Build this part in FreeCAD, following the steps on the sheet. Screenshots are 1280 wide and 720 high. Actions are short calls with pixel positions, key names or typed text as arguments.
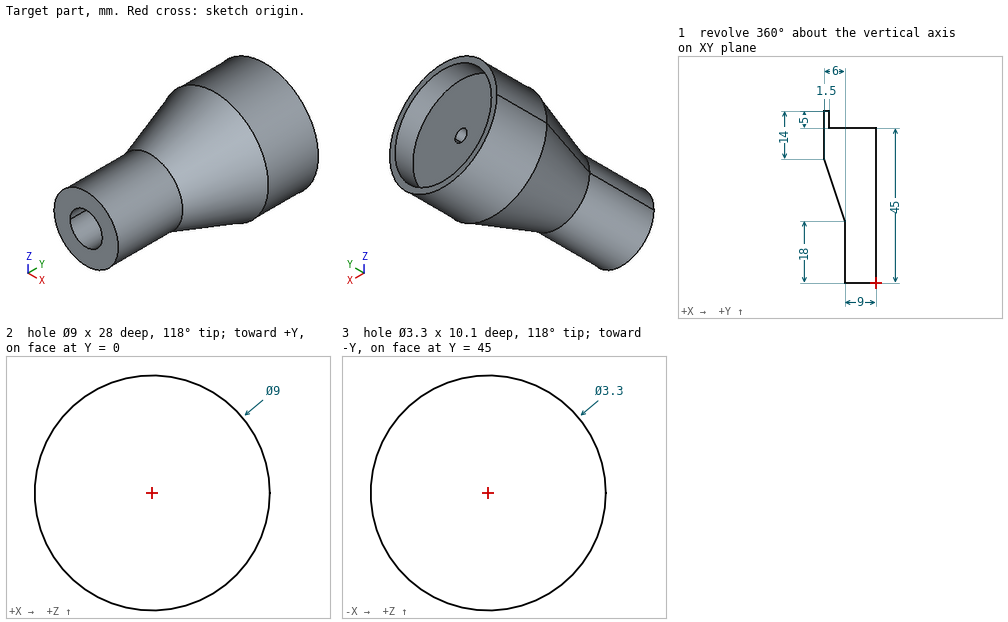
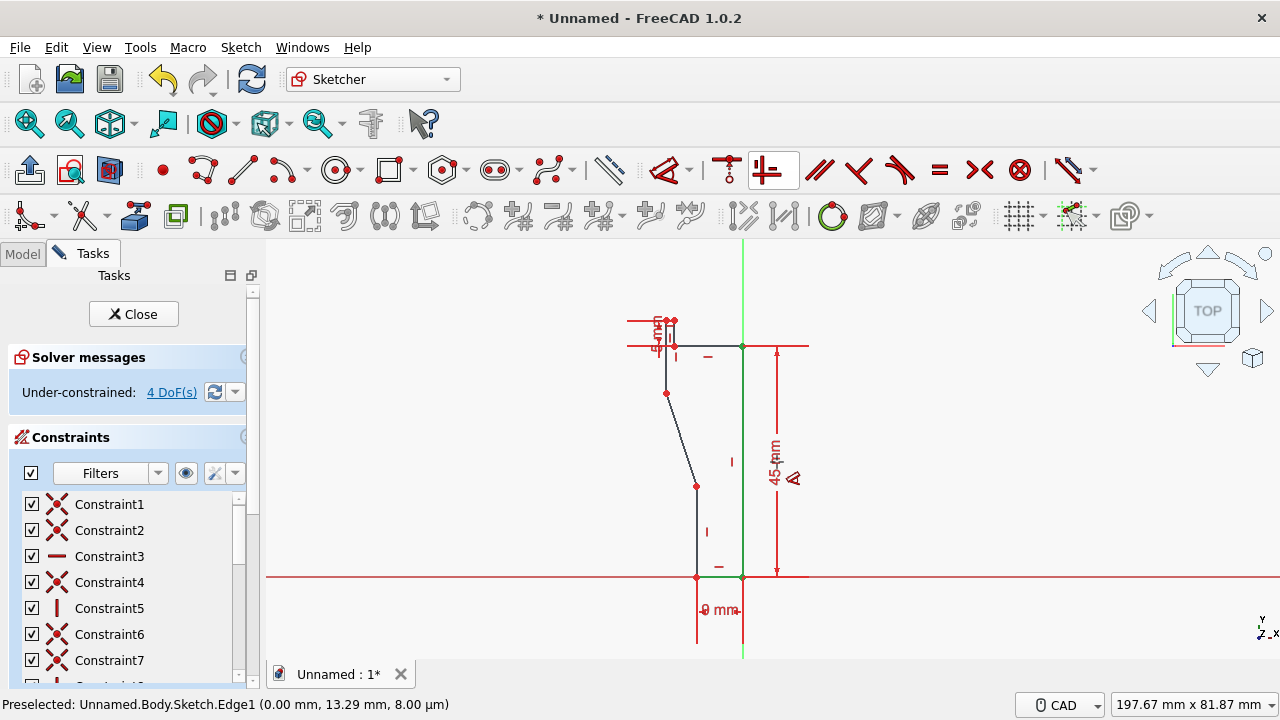
click(666, 371)
click(632, 357)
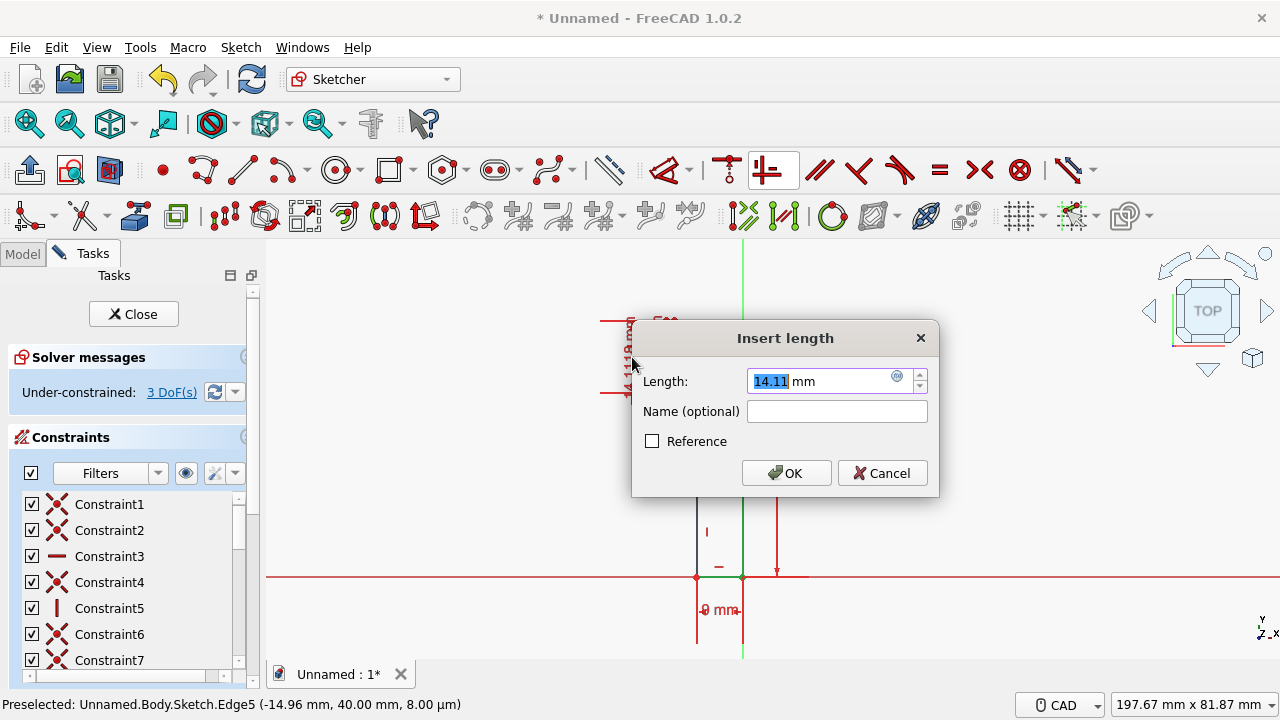
text(14)
key(Return)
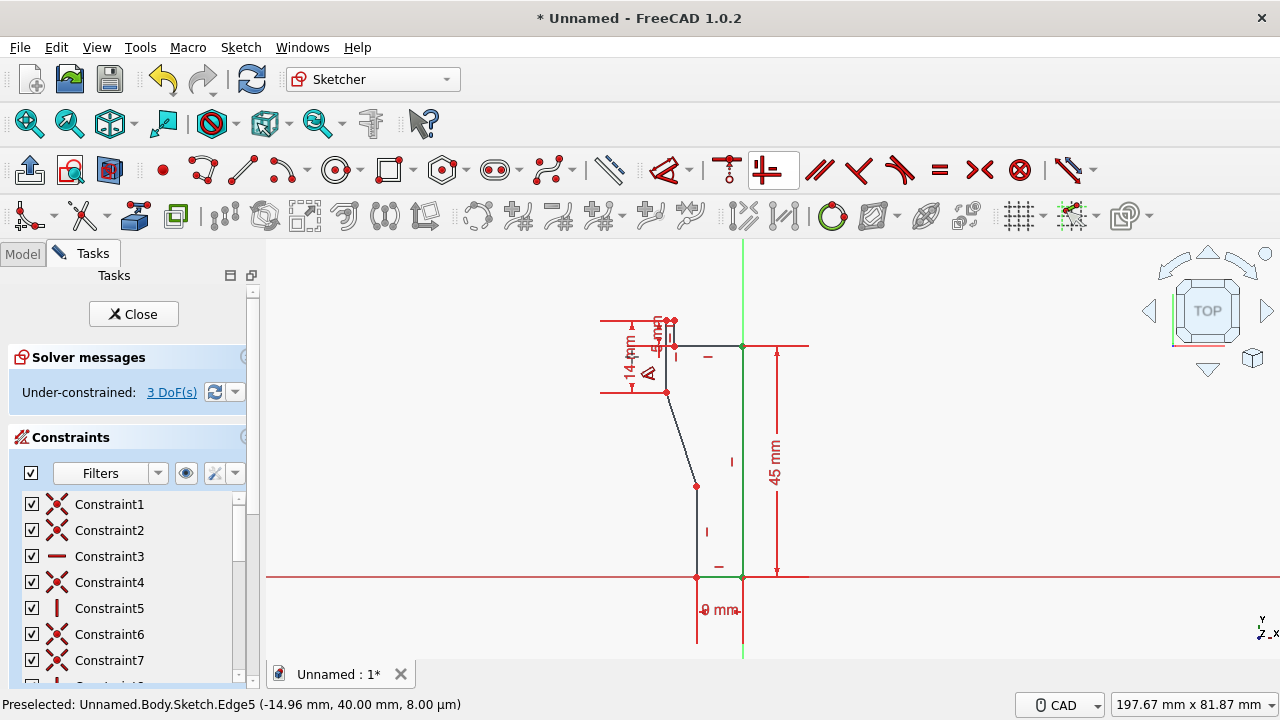
click(697, 513)
click(663, 532)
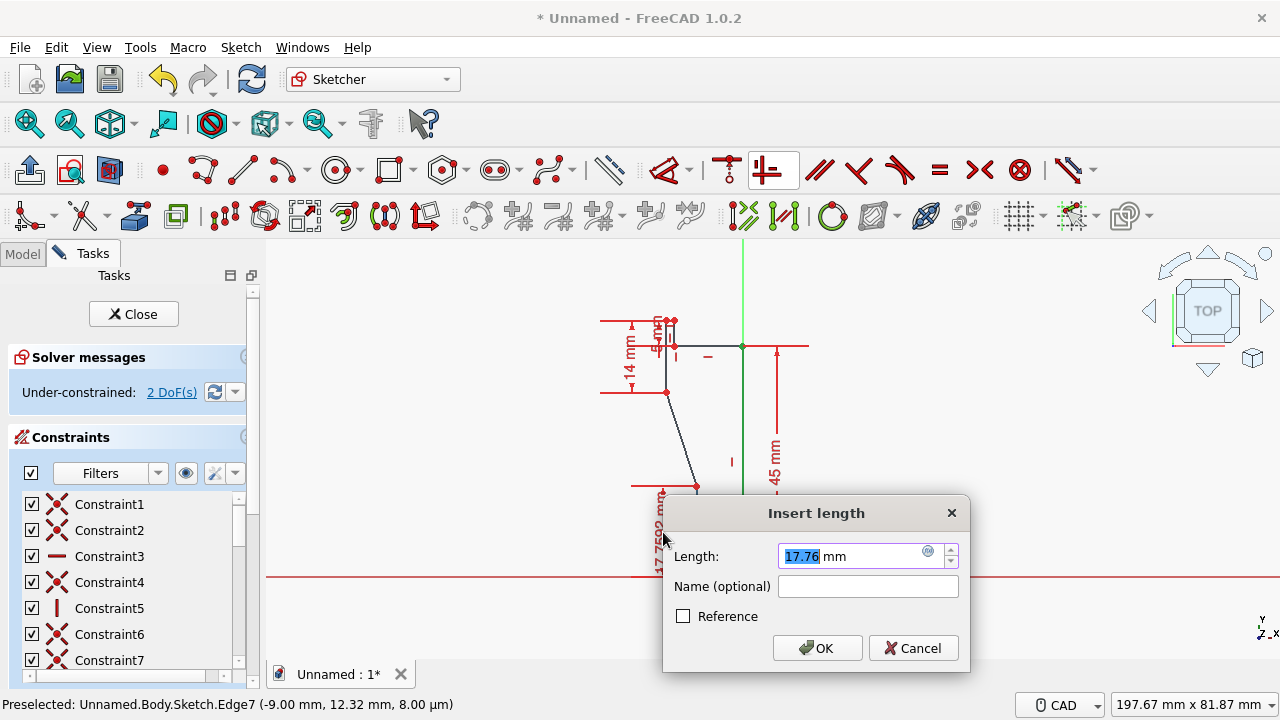
text(18)
key(Return)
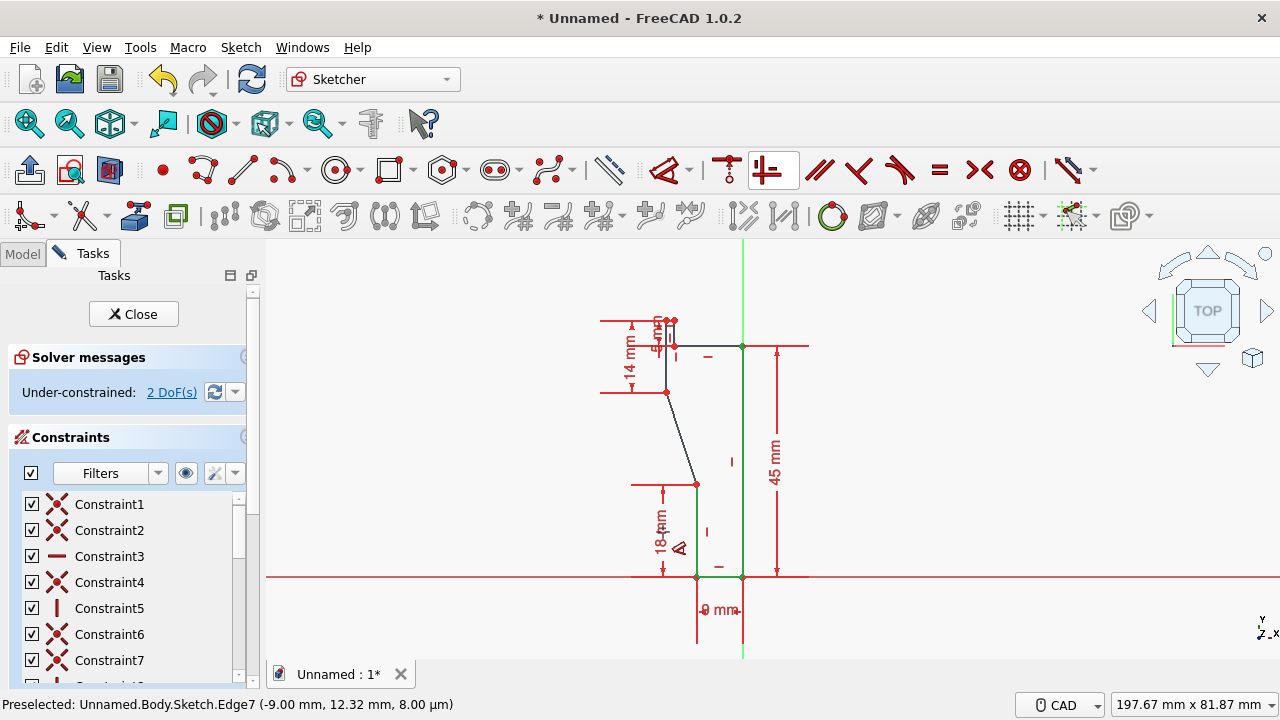
scroll(675, 420, up, 2)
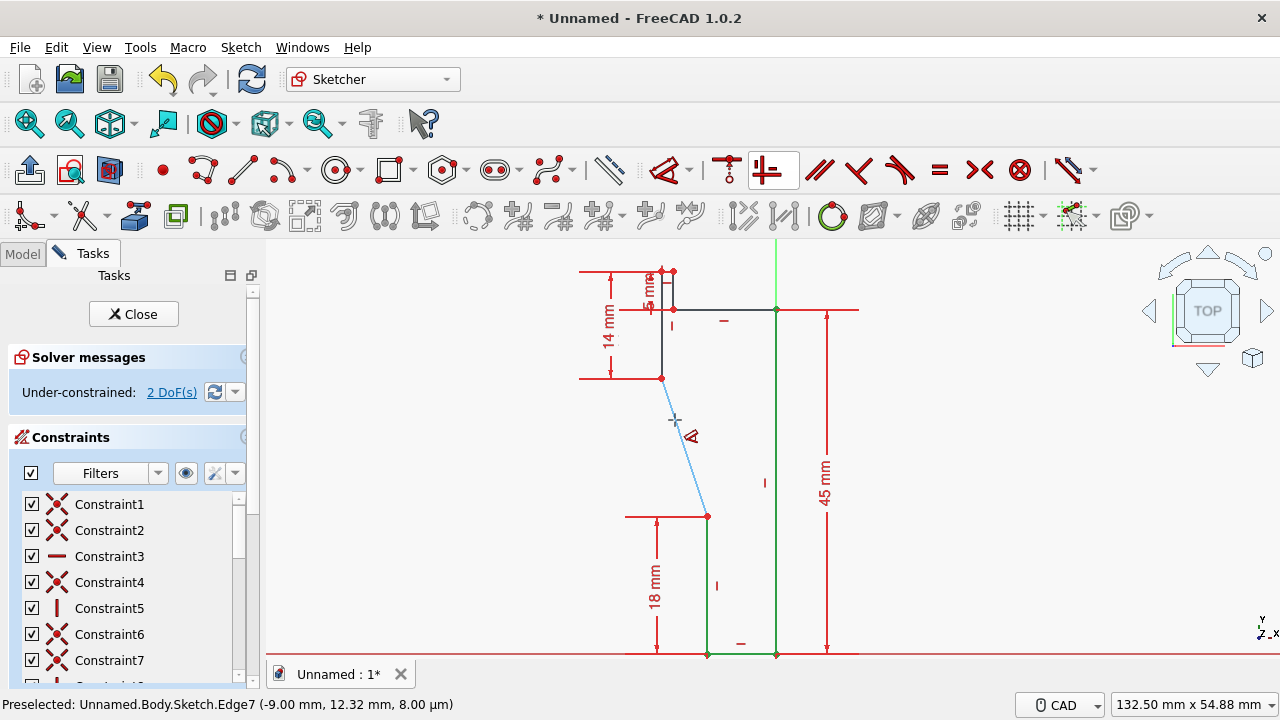
click(675, 420)
click(685, 345)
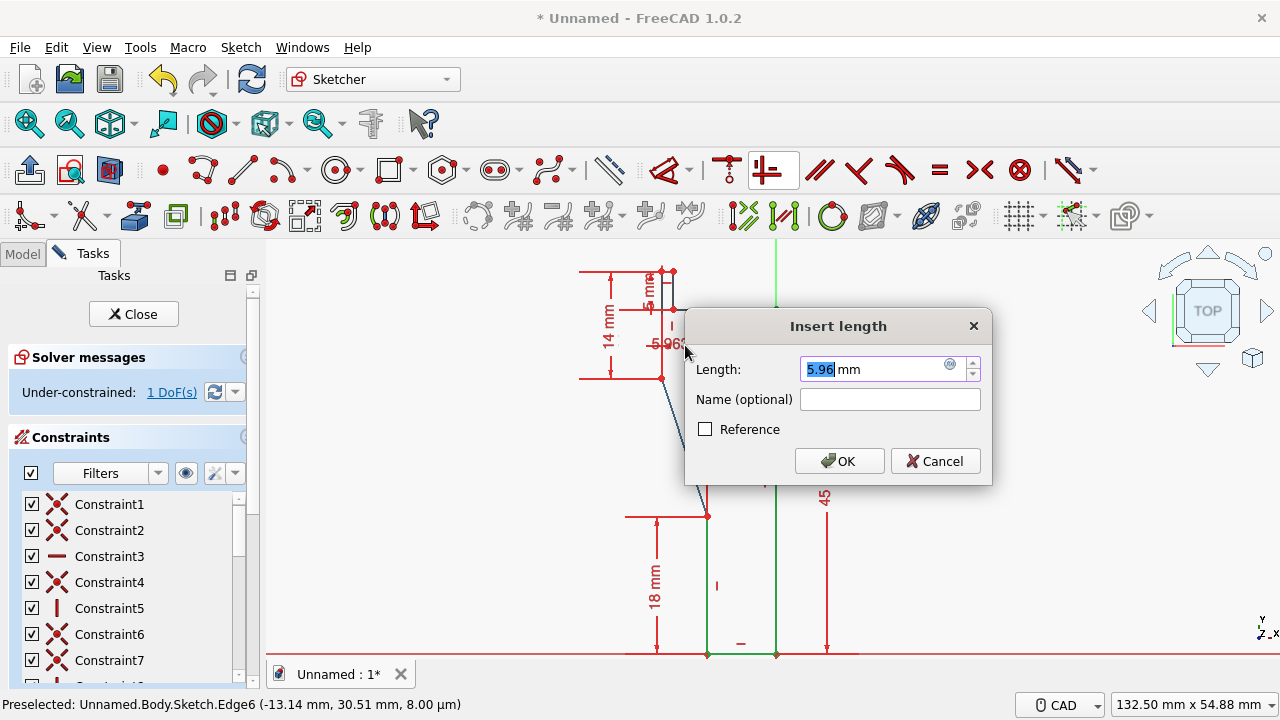
text(6)
key(Return)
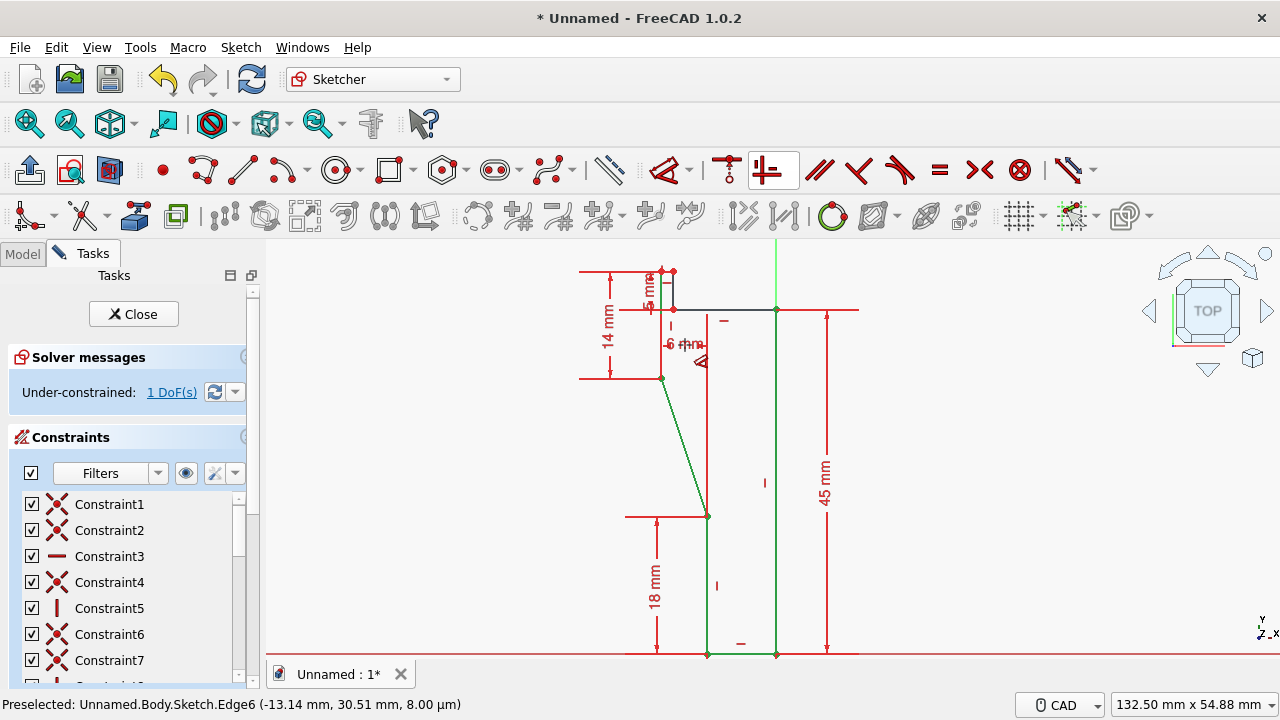
scroll(667, 272, up, 7)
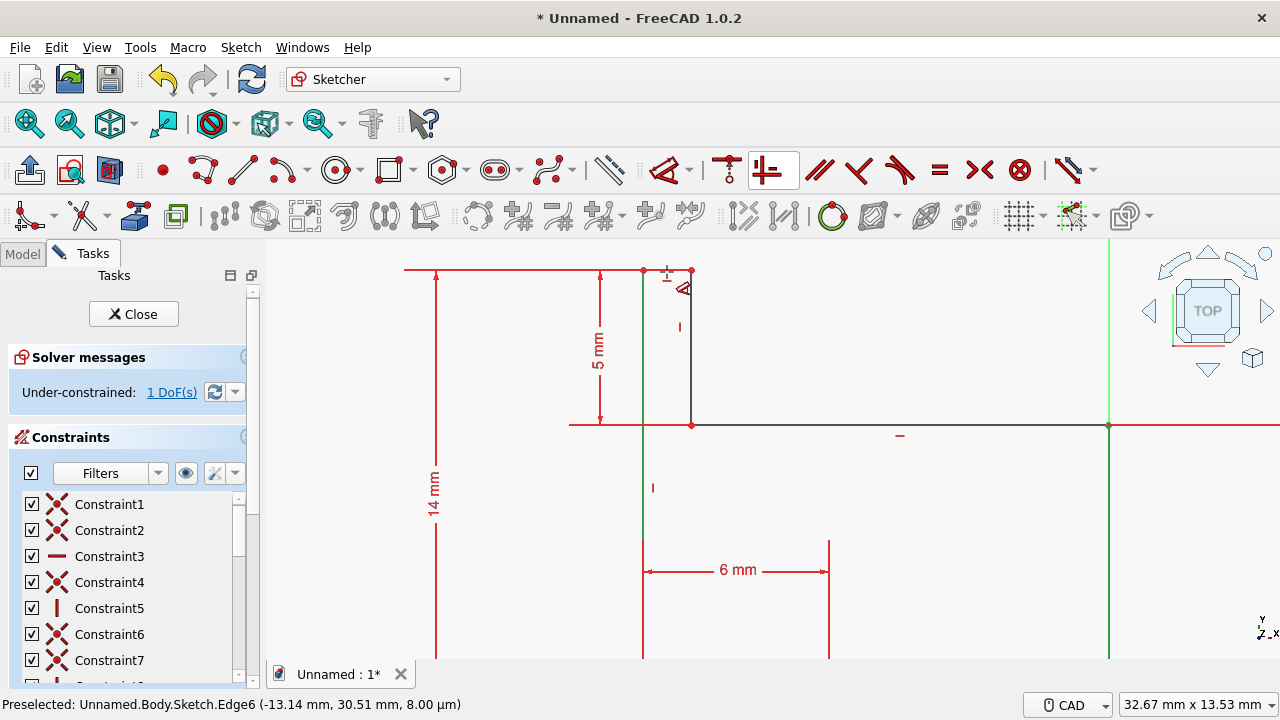
click(667, 270)
click(667, 304)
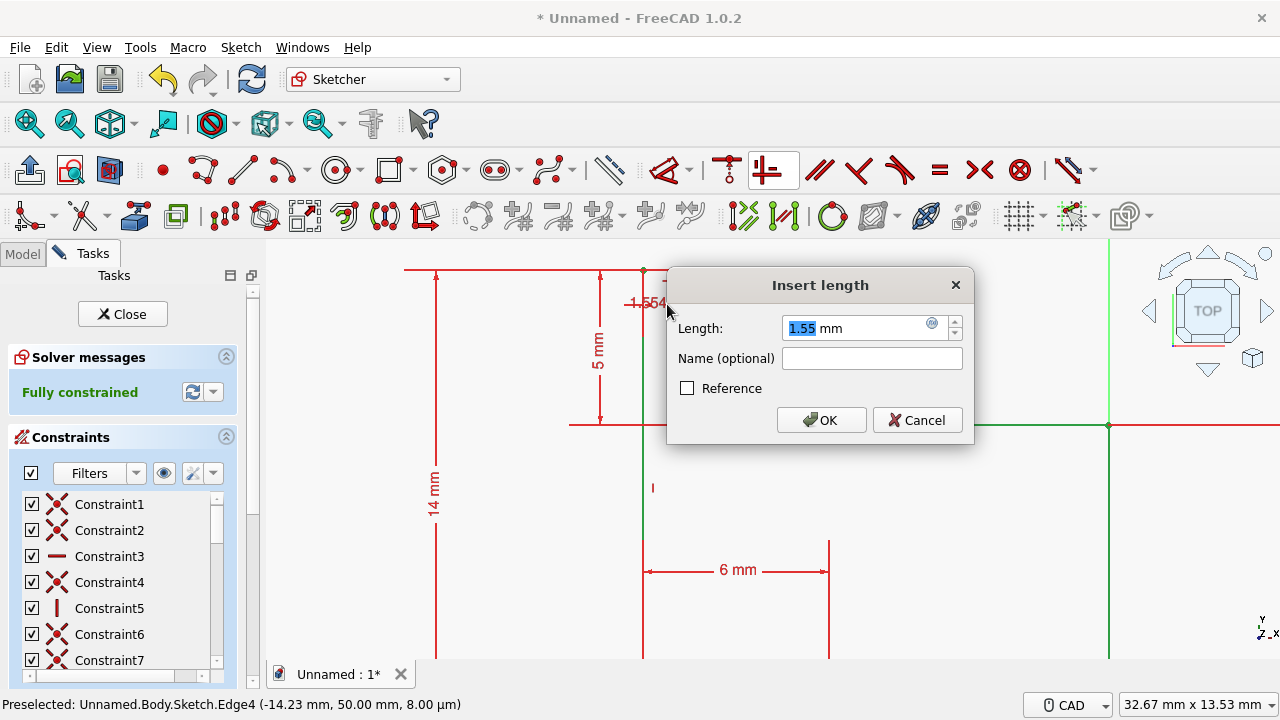
text(1.5)
key(Return)
key(Escape)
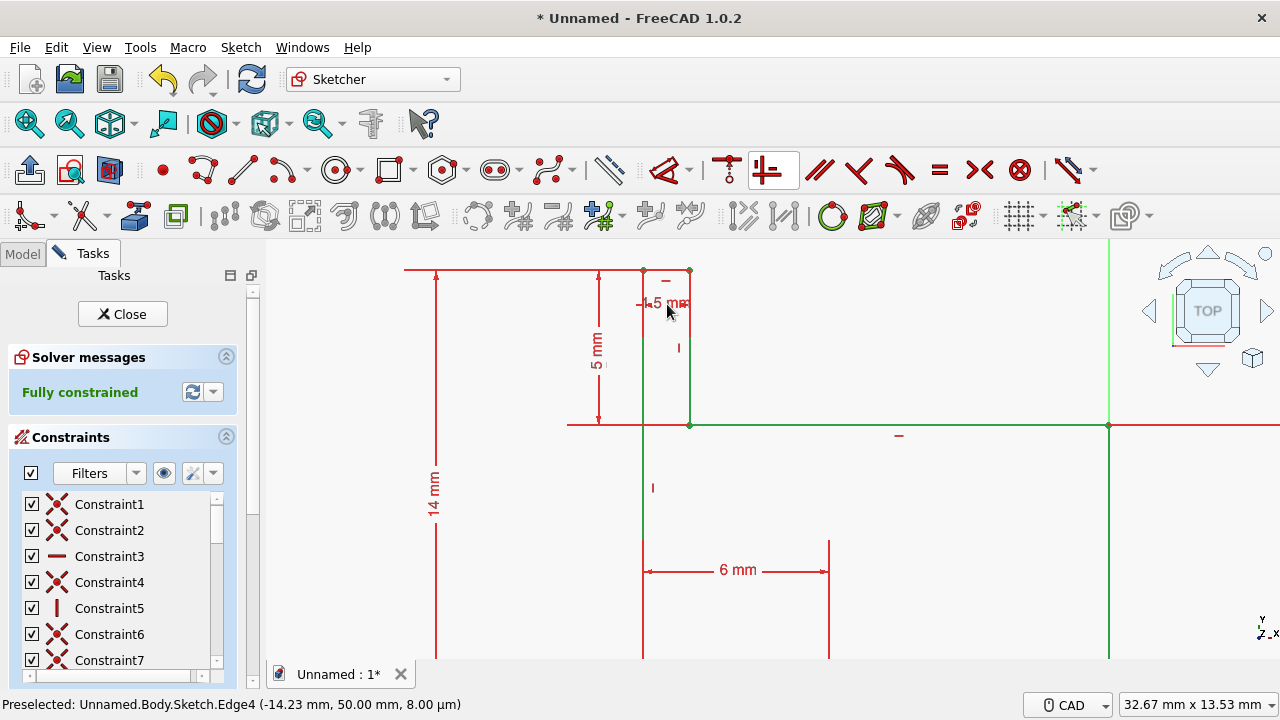
click(123, 314)